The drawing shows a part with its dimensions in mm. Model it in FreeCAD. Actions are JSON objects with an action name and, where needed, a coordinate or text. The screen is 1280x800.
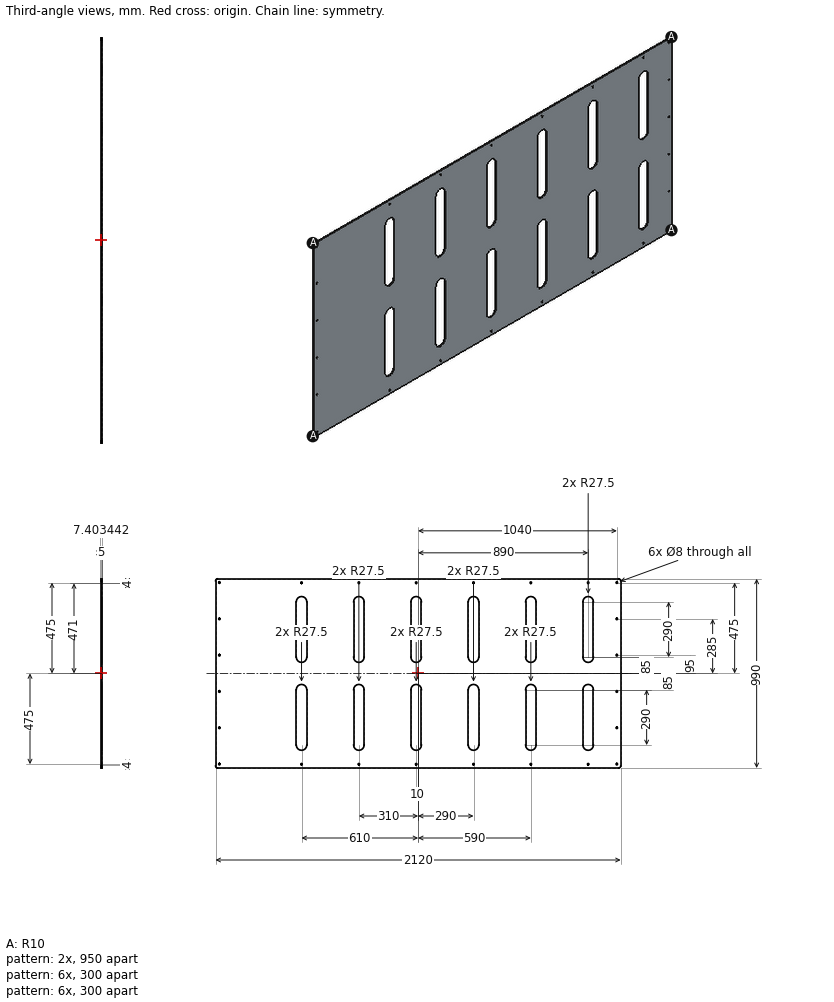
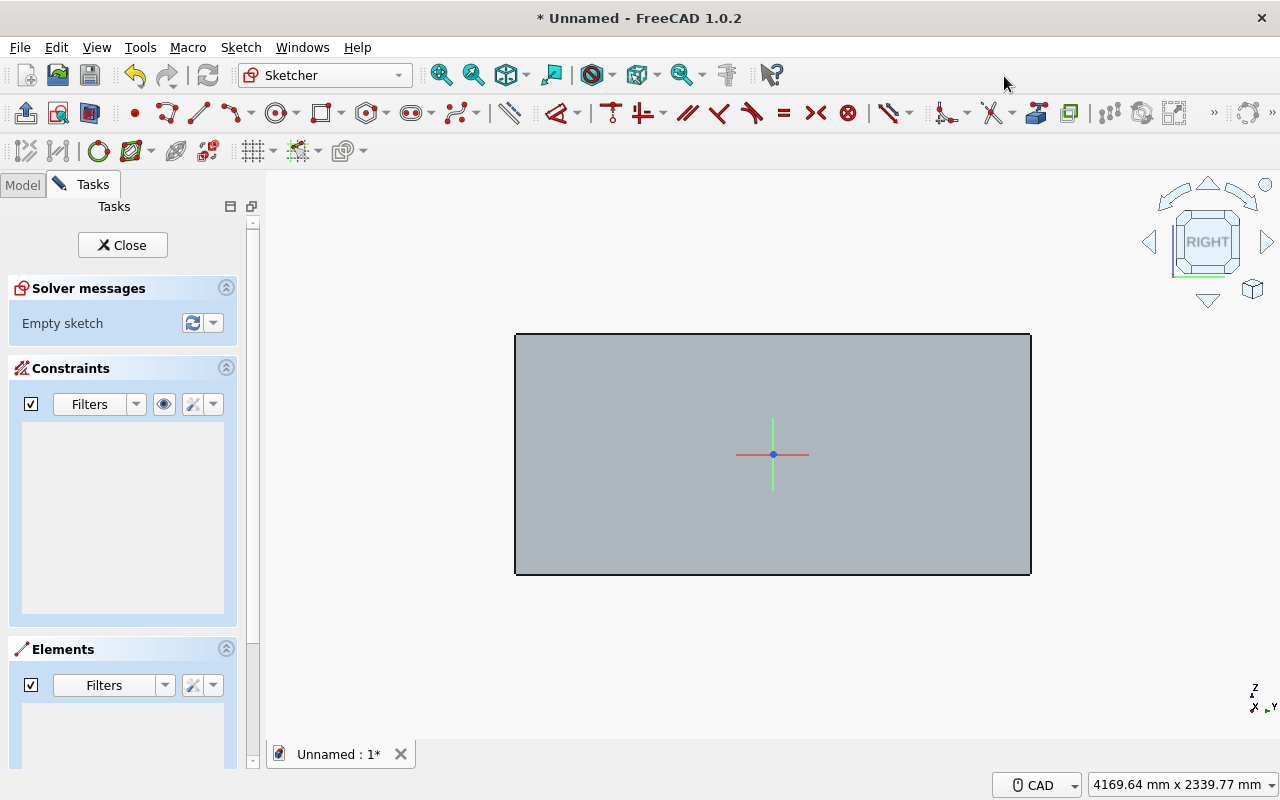
{"action": "scroll", "coordinate": [1115, 455], "scroll_direction": "up", "scroll_amount": 2}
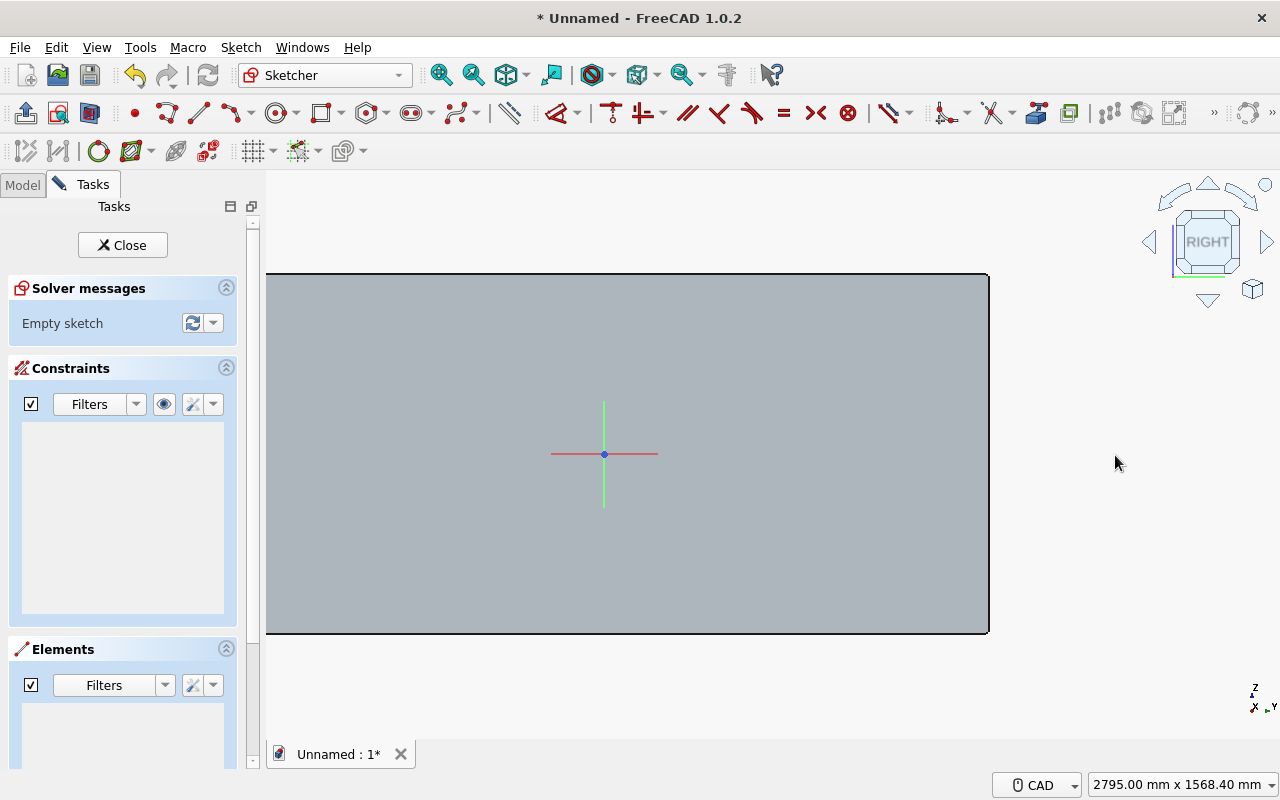
{"action": "key", "text": "g c"}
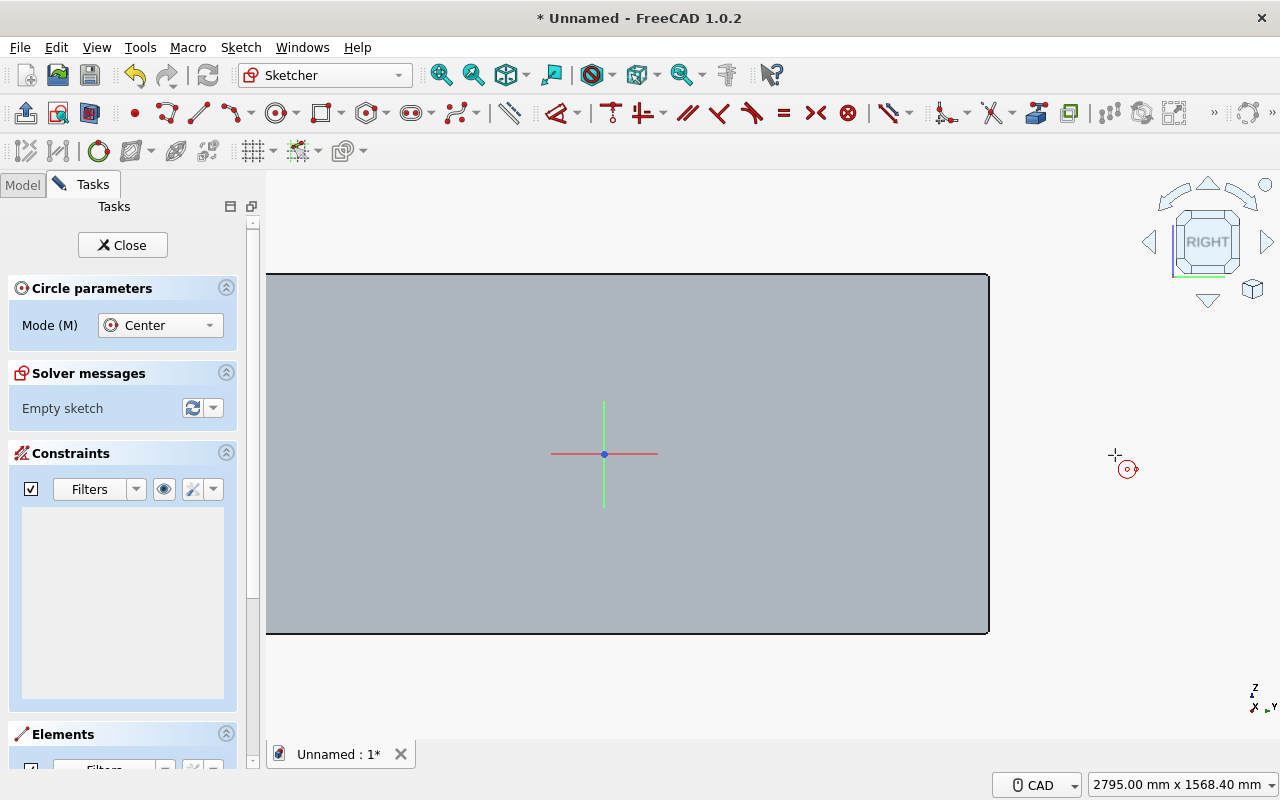
{"action": "scroll", "coordinate": [982, 282], "scroll_direction": "up", "scroll_amount": 14}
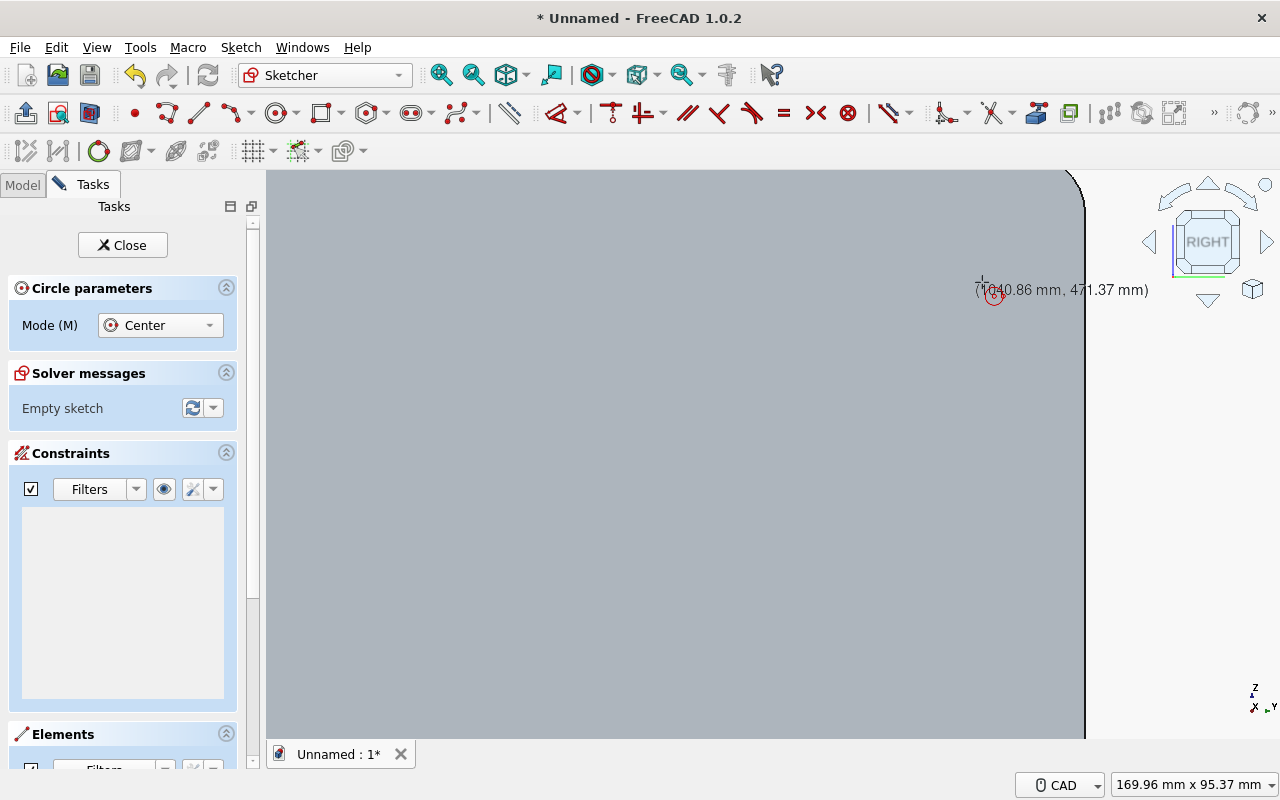
{"action": "scroll", "coordinate": [888, 283], "scroll_direction": "down", "scroll_amount": 14}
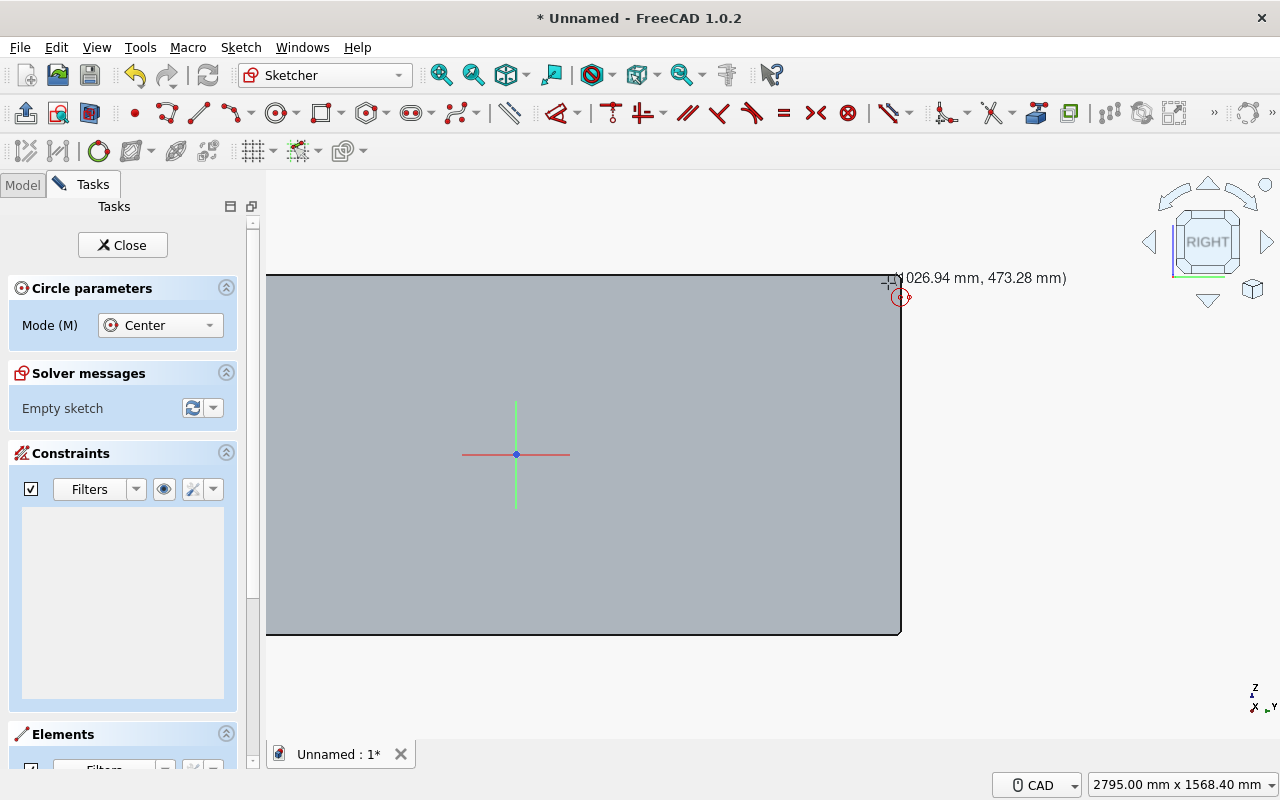
{"action": "left_click", "coordinate": [893, 283]}
{"action": "mouse_move", "coordinate": [894, 282]}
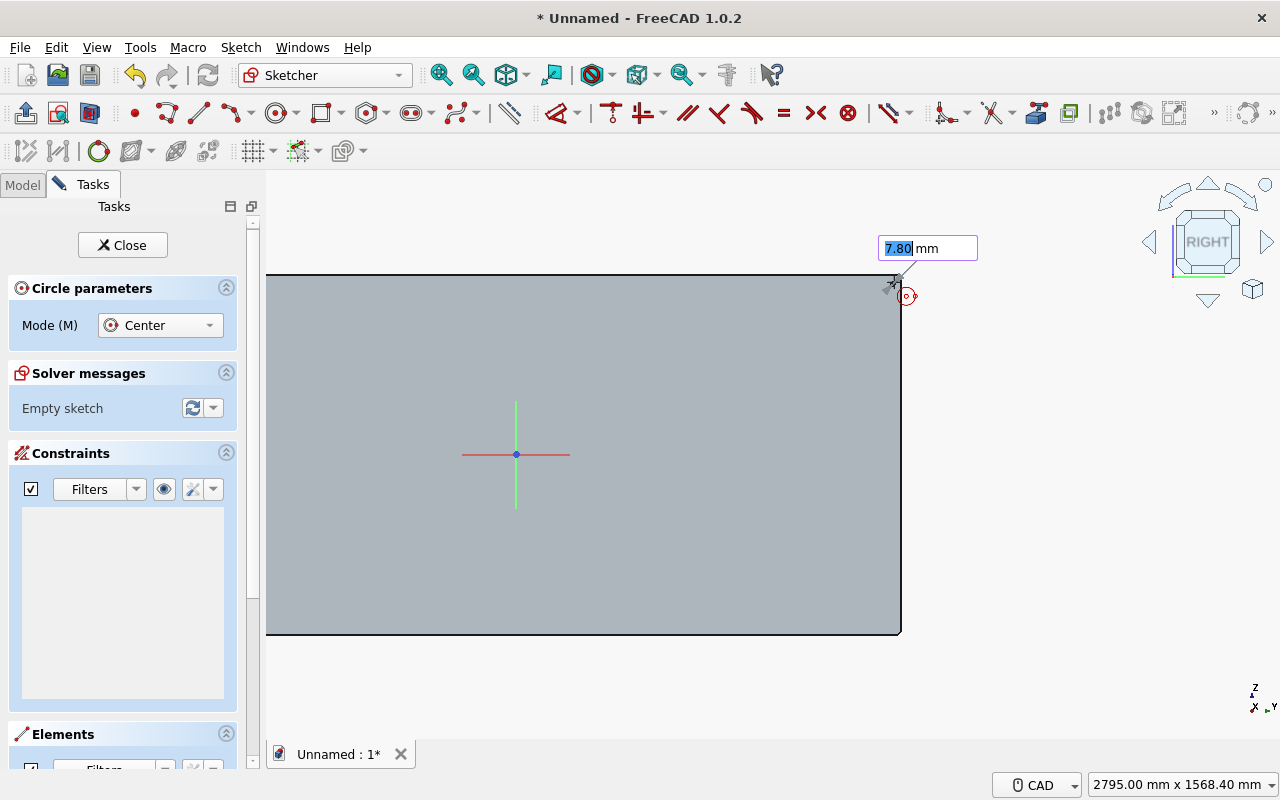
{"action": "type", "text": "8"}
{"action": "key", "text": "Return"}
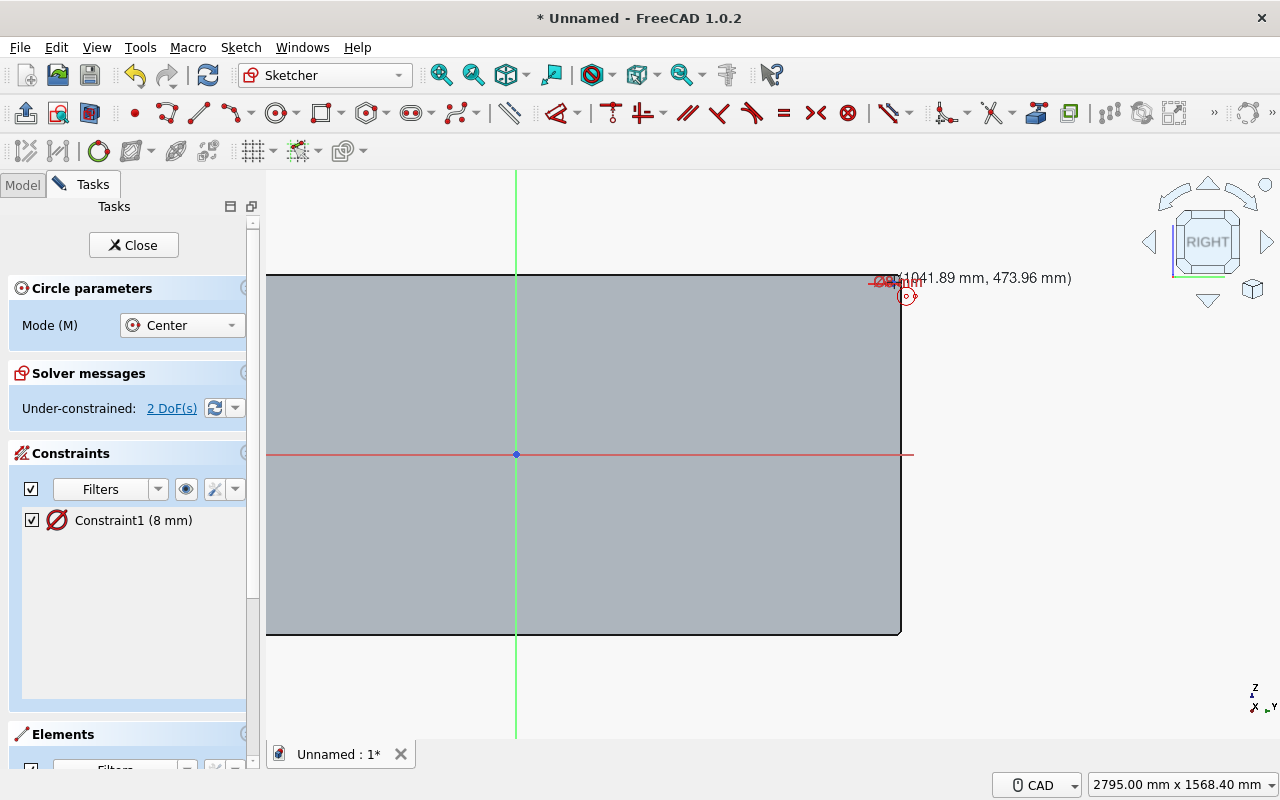
{"action": "scroll", "coordinate": [893, 352], "scroll_direction": "up", "scroll_amount": 14}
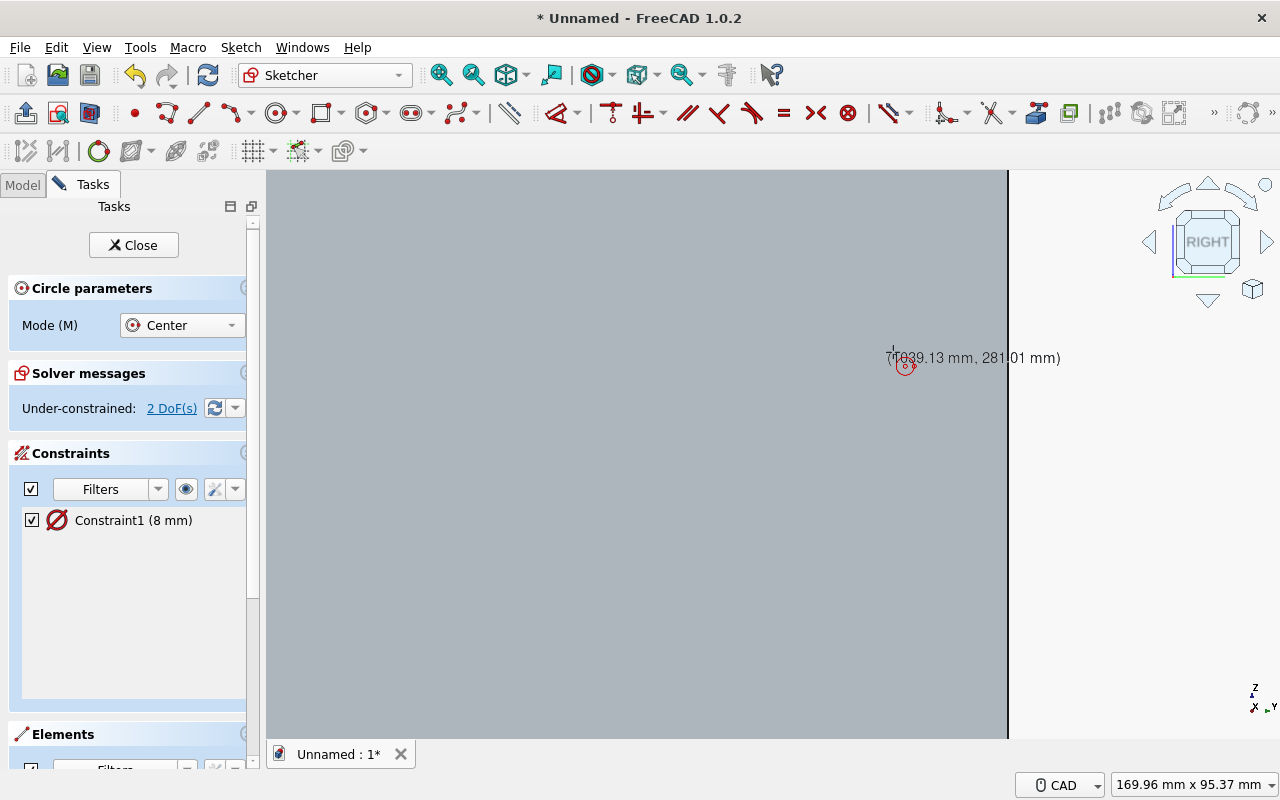
{"action": "scroll", "coordinate": [893, 352], "scroll_direction": "down", "scroll_amount": 14}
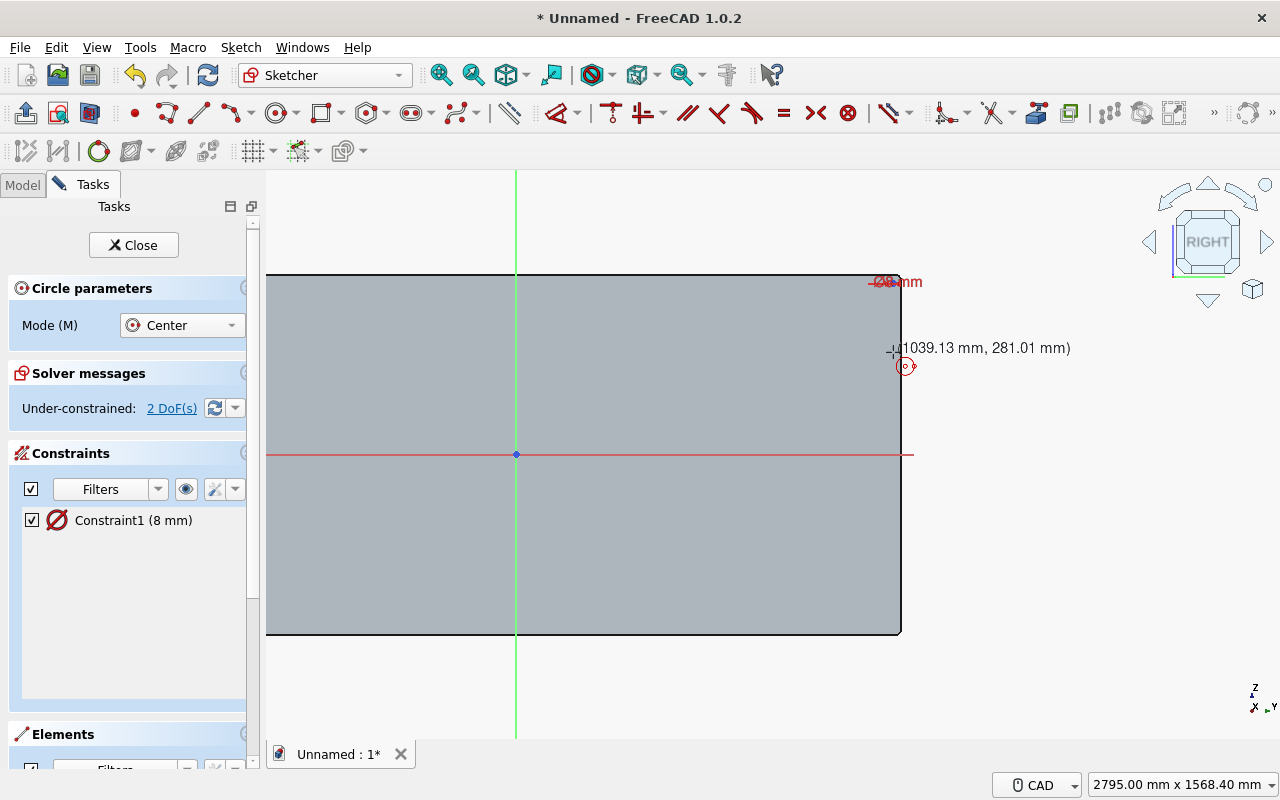
{"action": "left_click", "coordinate": [893, 352]}
{"action": "mouse_move", "coordinate": [894, 351]}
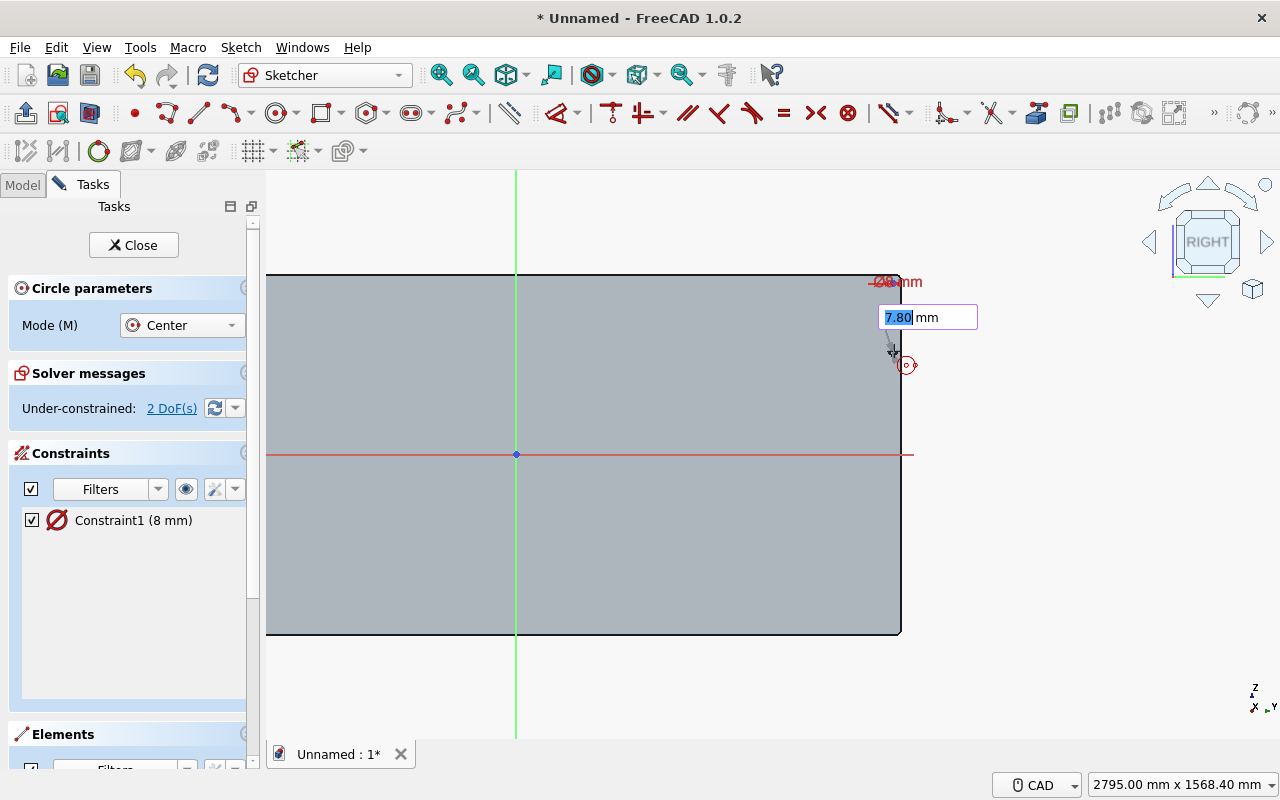
{"action": "type", "text": "8"}
{"action": "key", "text": "Return"}